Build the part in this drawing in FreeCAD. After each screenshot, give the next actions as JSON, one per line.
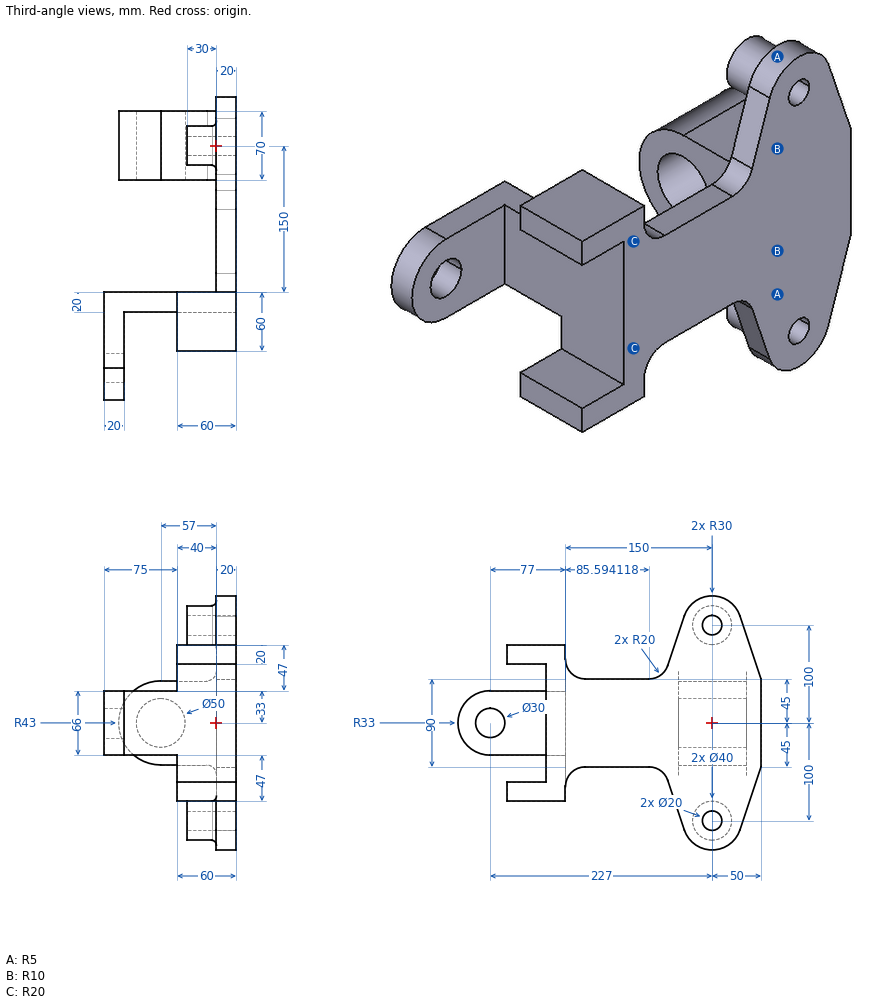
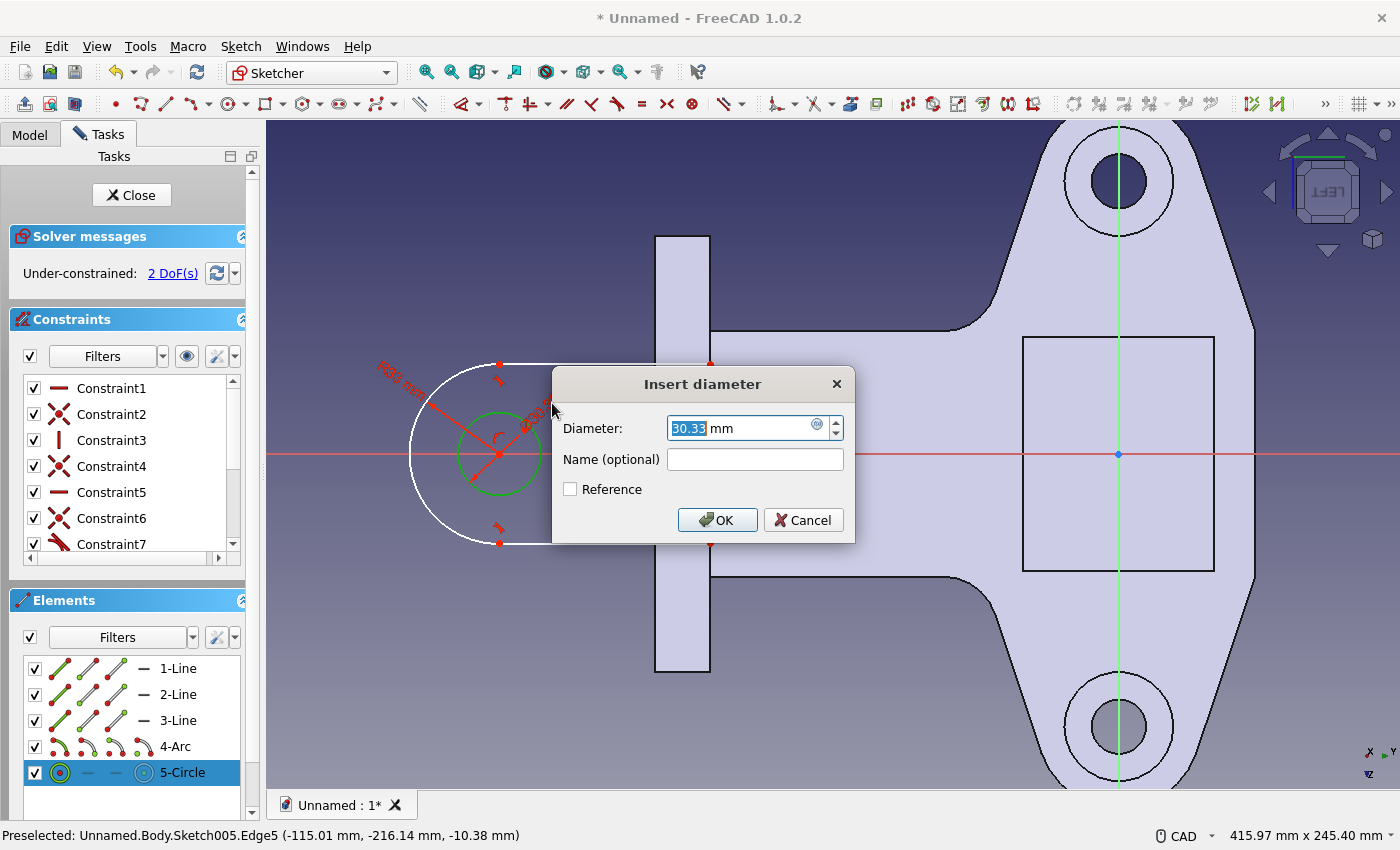
{"action": "type", "text": "30"}
{"action": "key", "text": "Return"}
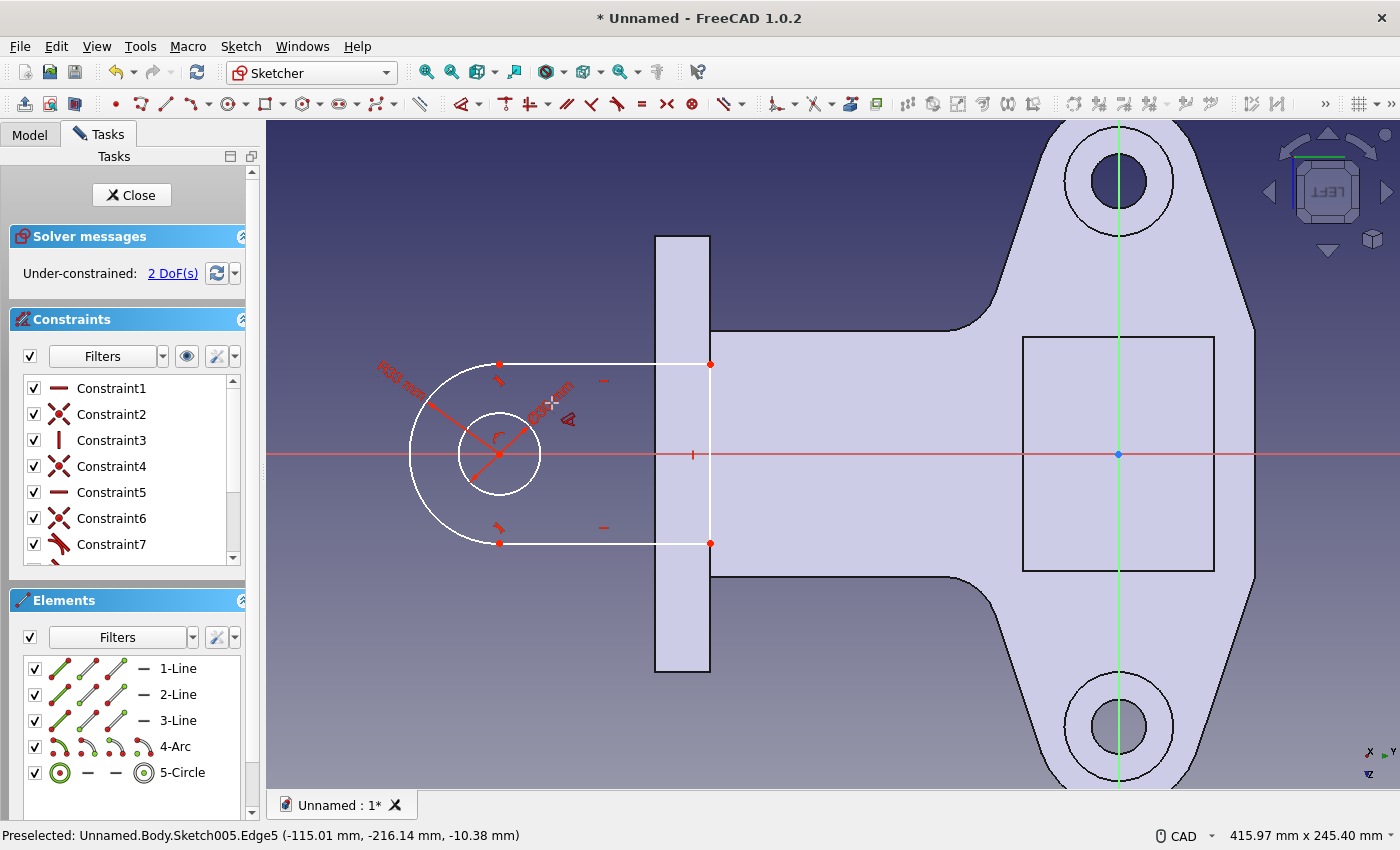
{"action": "left_click", "coordinate": [563, 544]}
{"action": "left_click", "coordinate": [605, 578]}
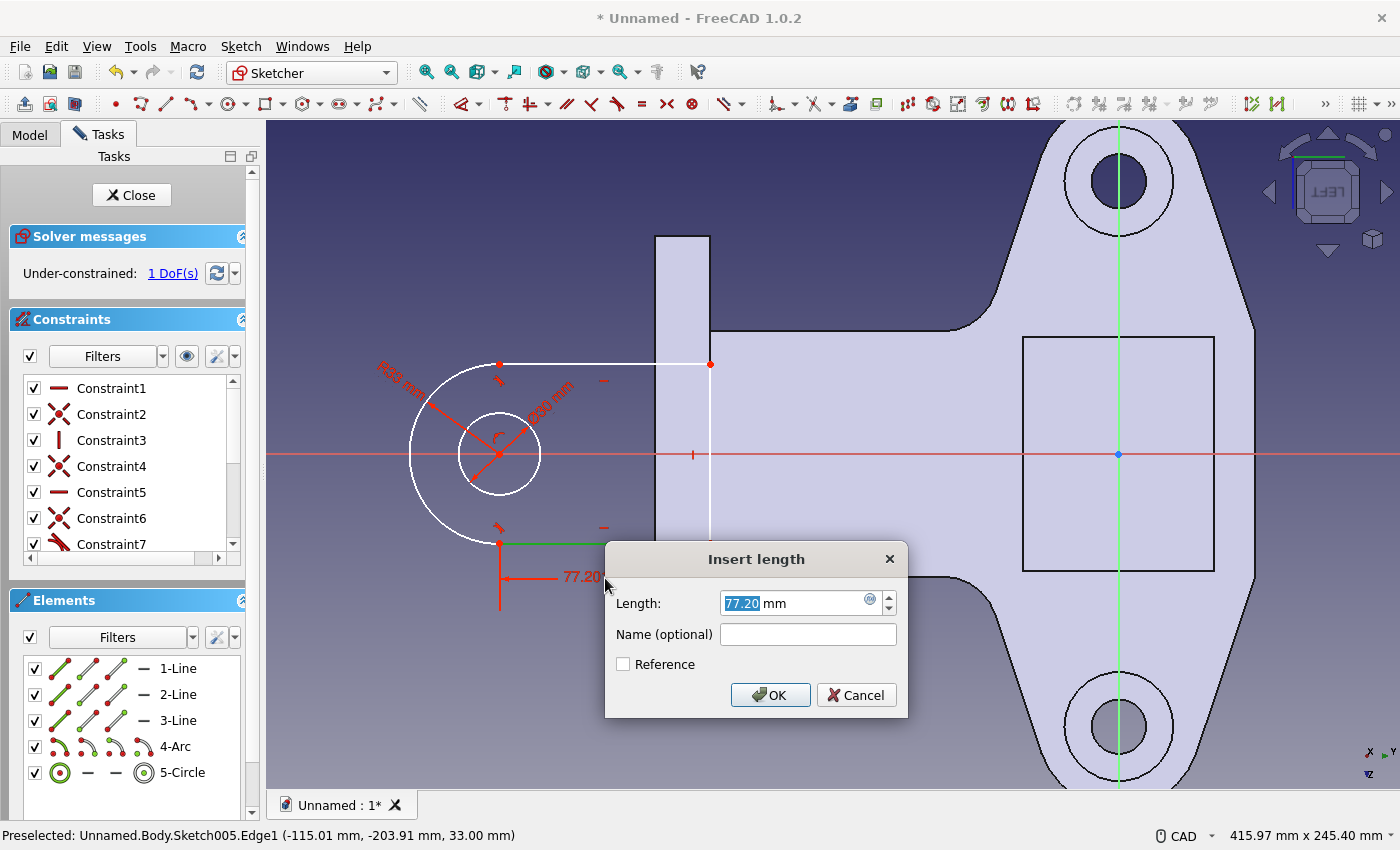
{"action": "type", "text": "77"}
{"action": "key", "text": "Return"}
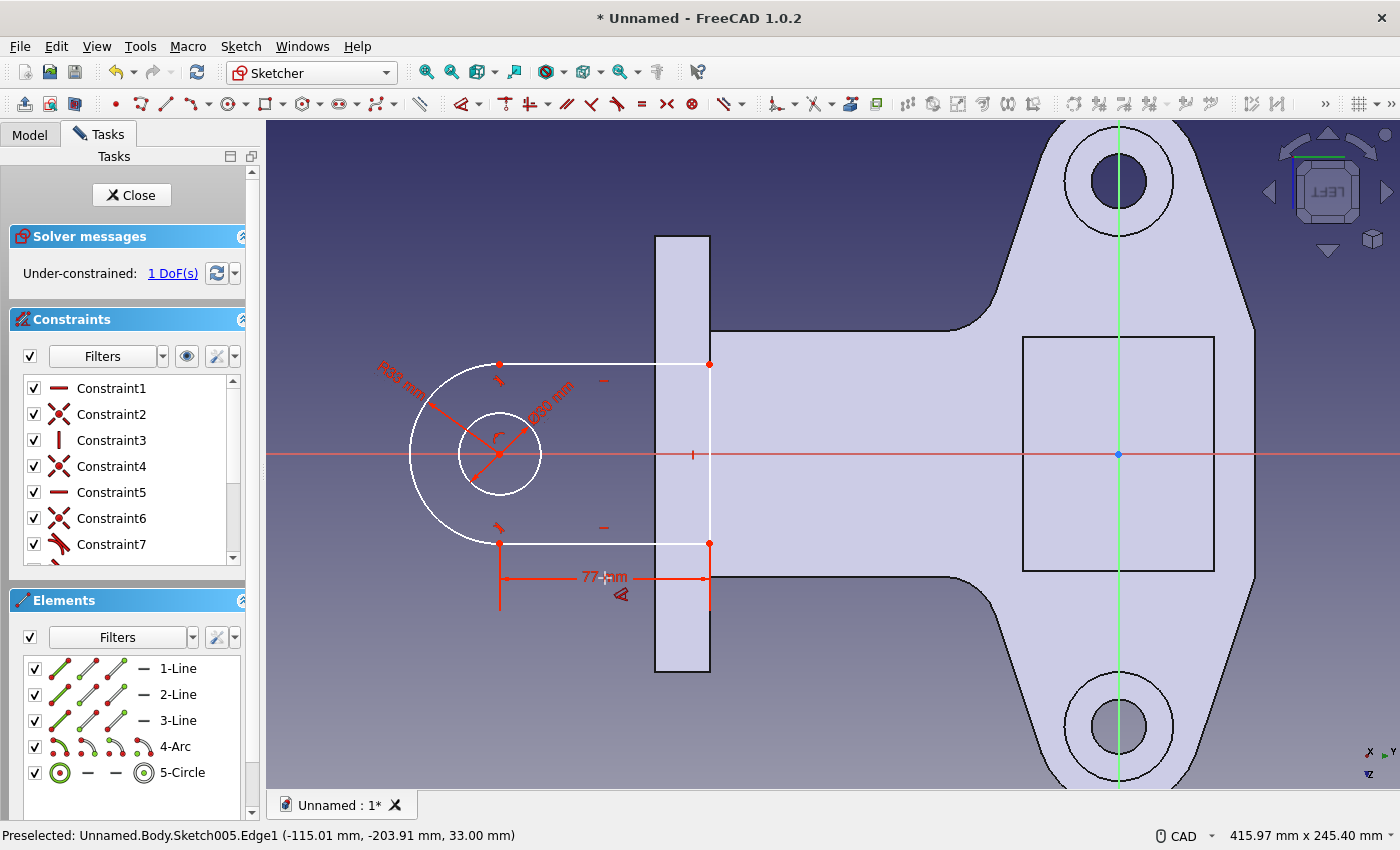
{"action": "left_click", "coordinate": [500, 454]}
{"action": "left_click", "coordinate": [809, 488]}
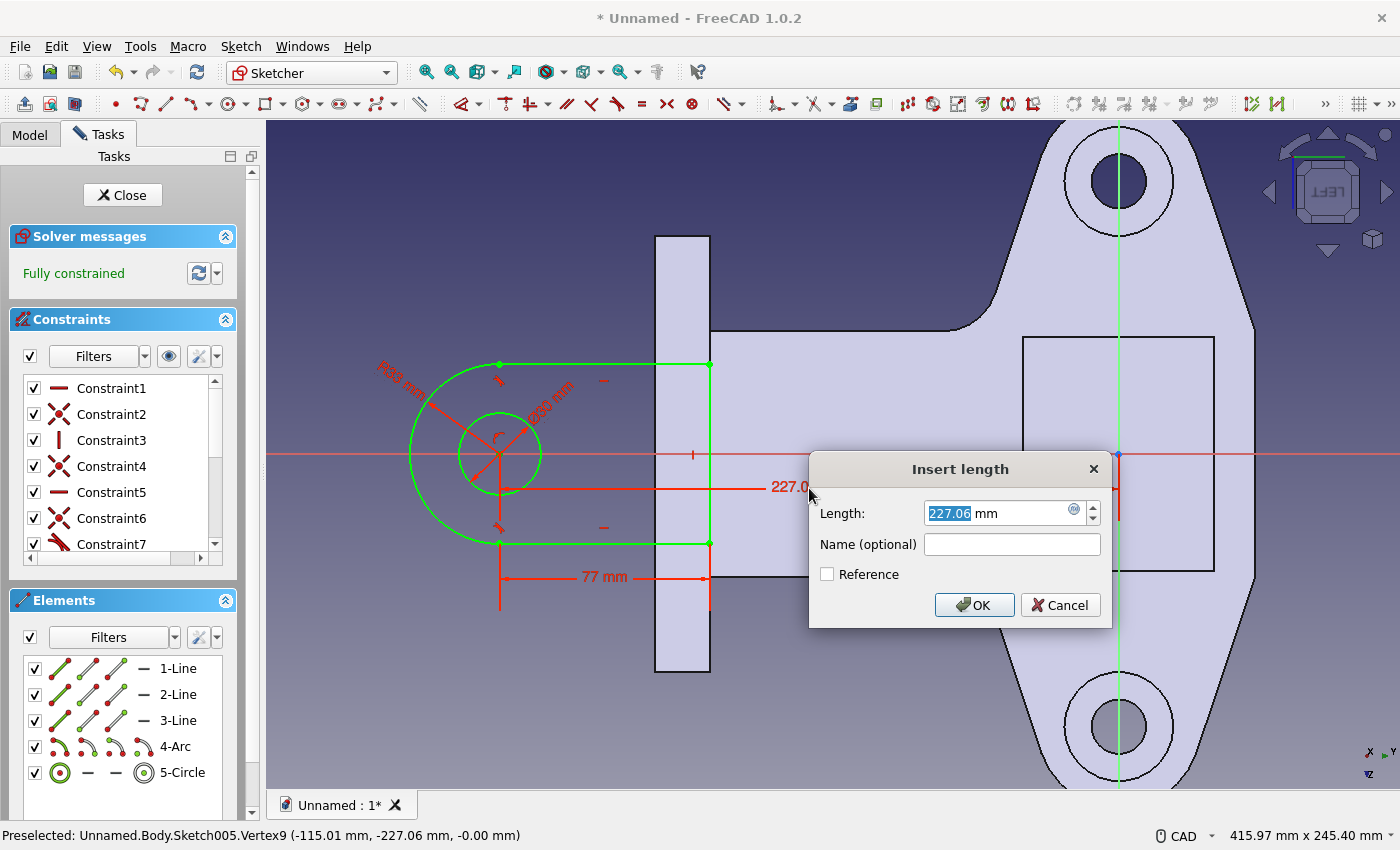
{"action": "type", "text": "227"}
{"action": "key", "text": "Return"}
{"action": "key", "text": "Escape"}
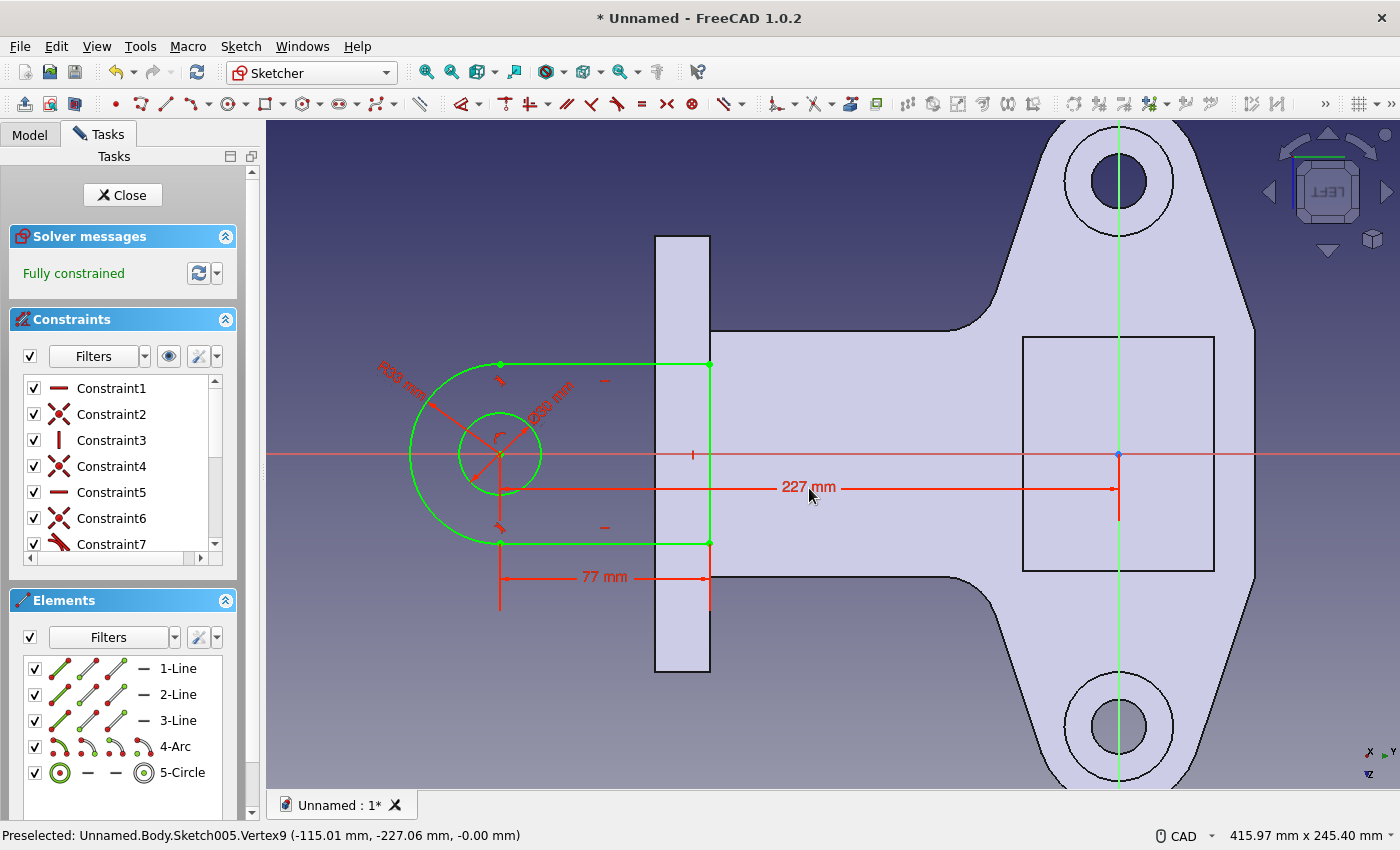
{"action": "left_click", "coordinate": [123, 195]}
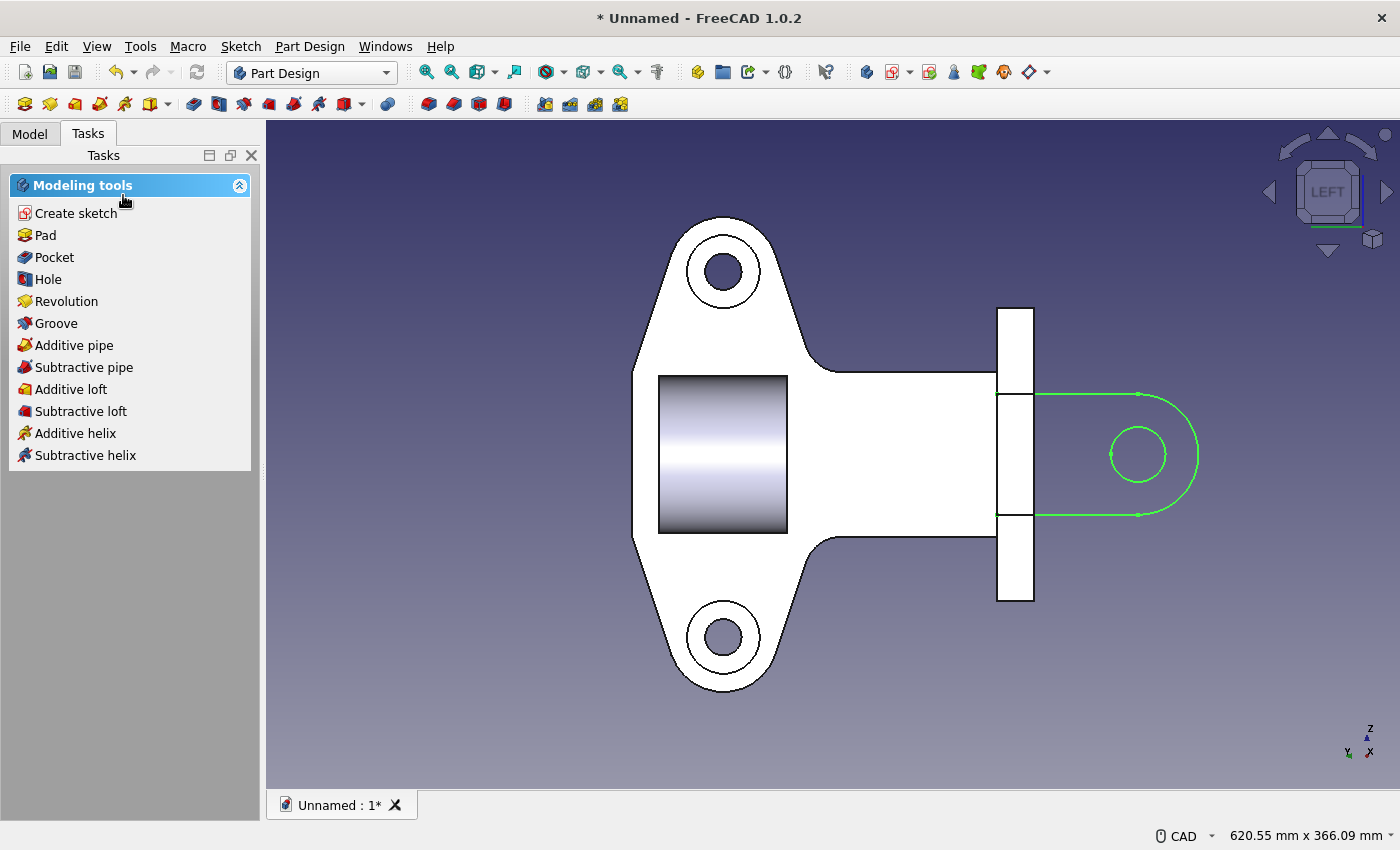
{"action": "left_click", "coordinate": [25, 104]}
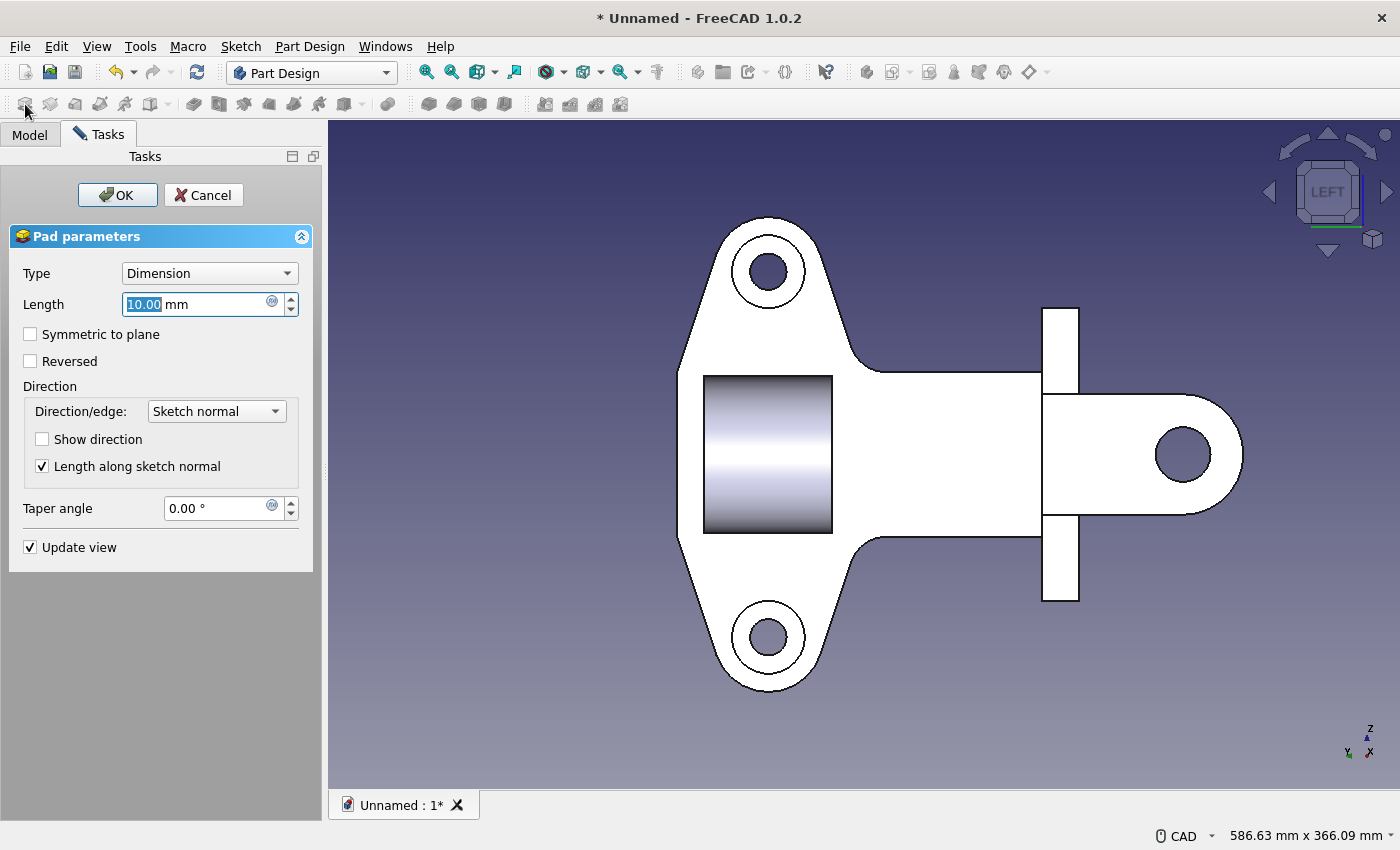
{"action": "type", "text": "20"}
{"action": "key", "text": "Tab"}